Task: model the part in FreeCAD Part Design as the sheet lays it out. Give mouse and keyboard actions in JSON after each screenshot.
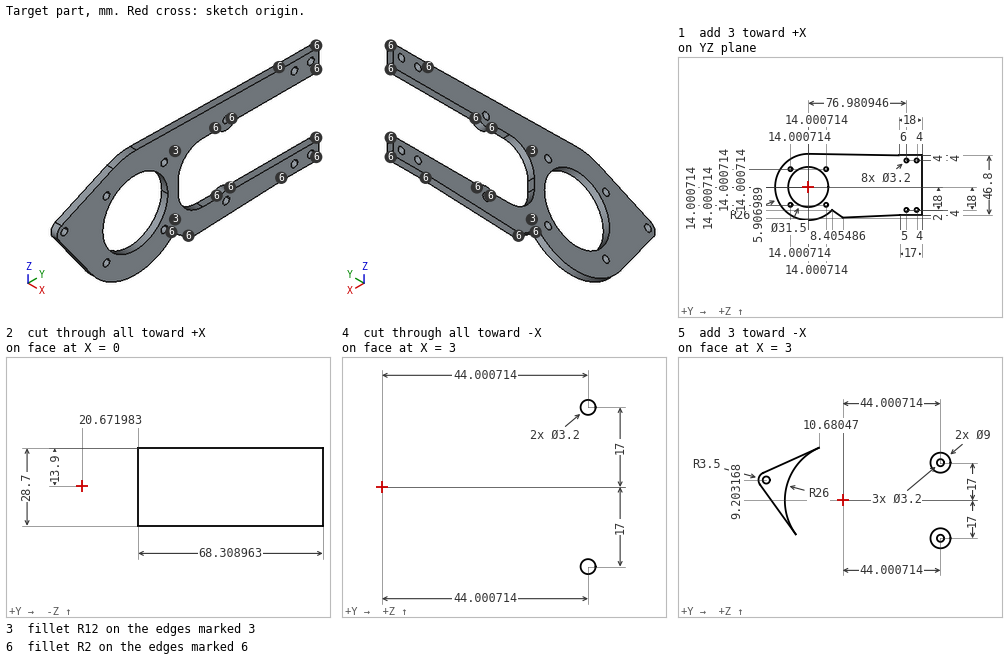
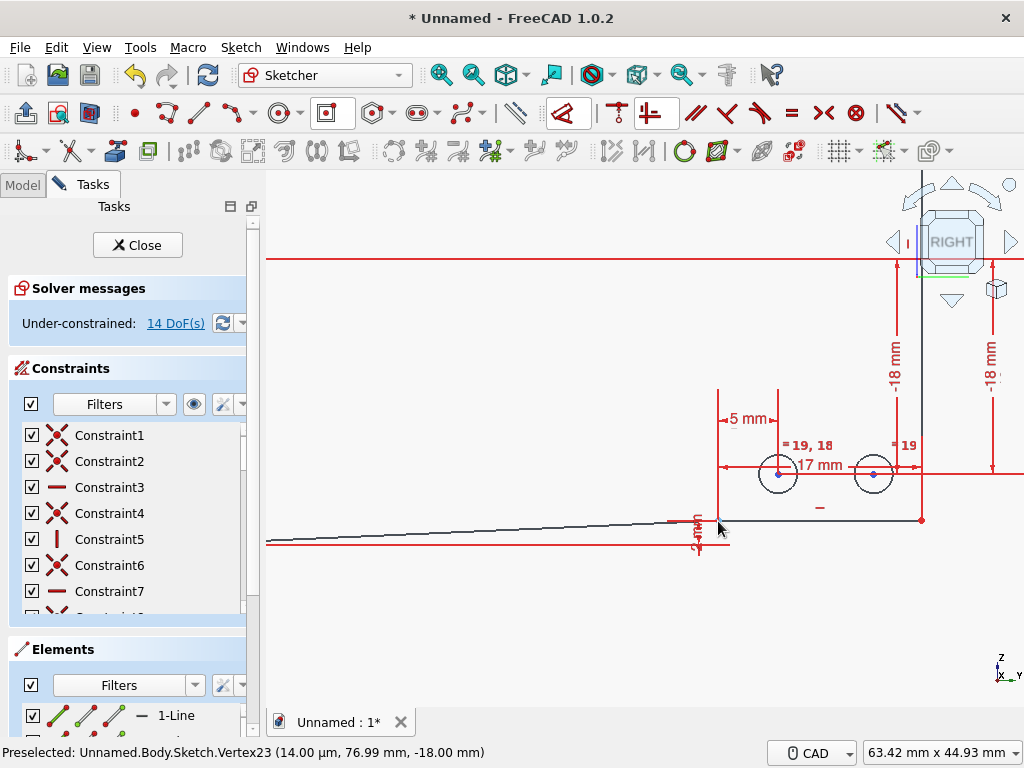
{"action": "left_click", "coordinate": [718, 521]}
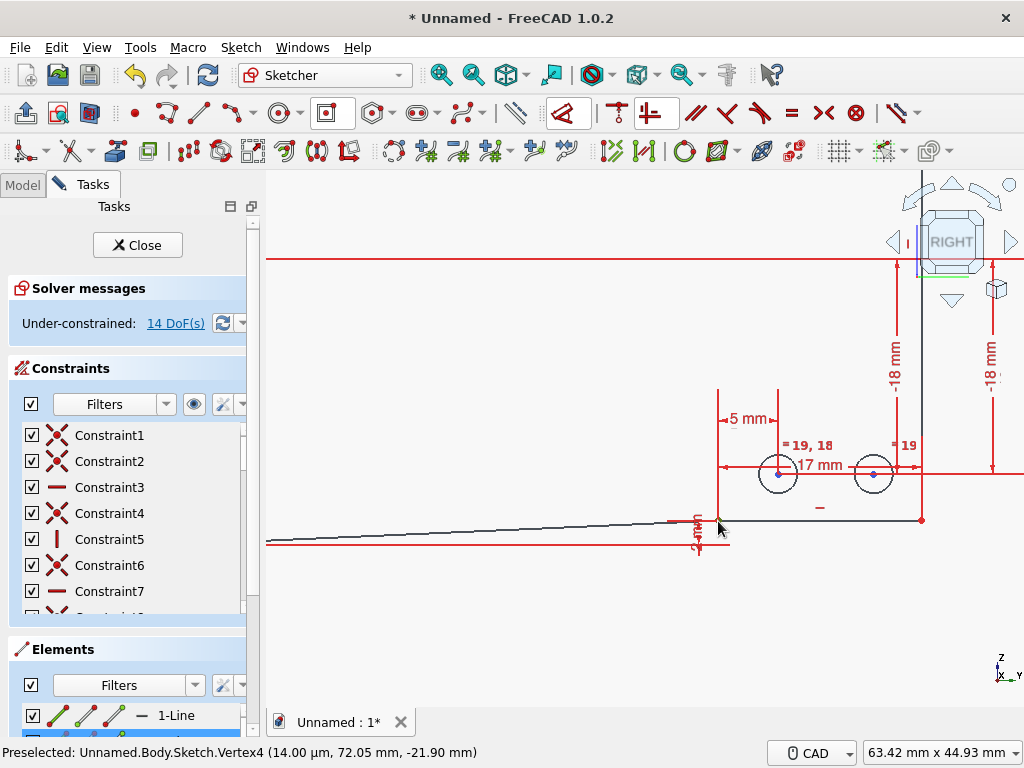
{"action": "left_click", "coordinate": [778, 474]}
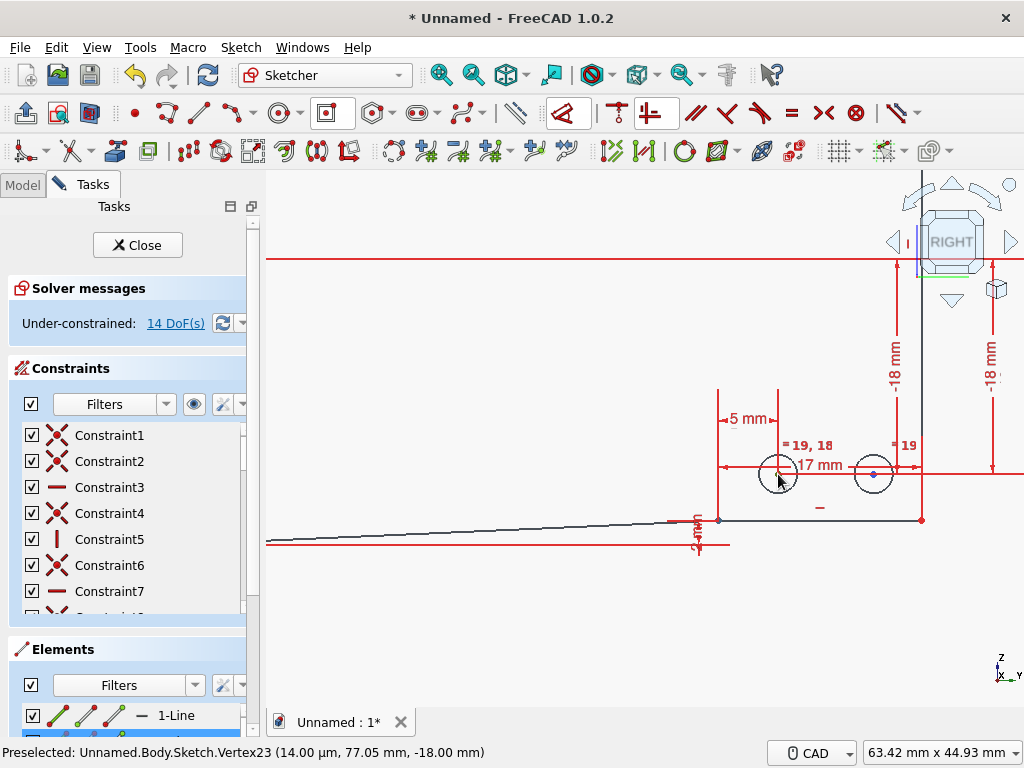
{"action": "left_click", "coordinate": [586, 114]}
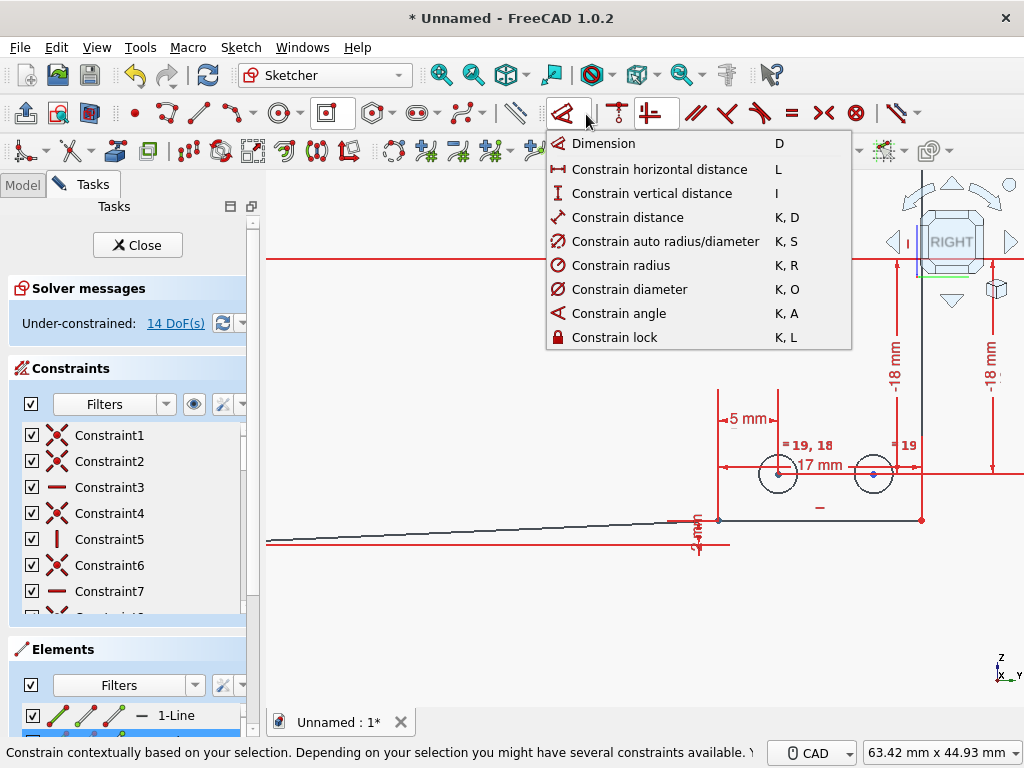
{"action": "left_click", "coordinate": [699, 193]}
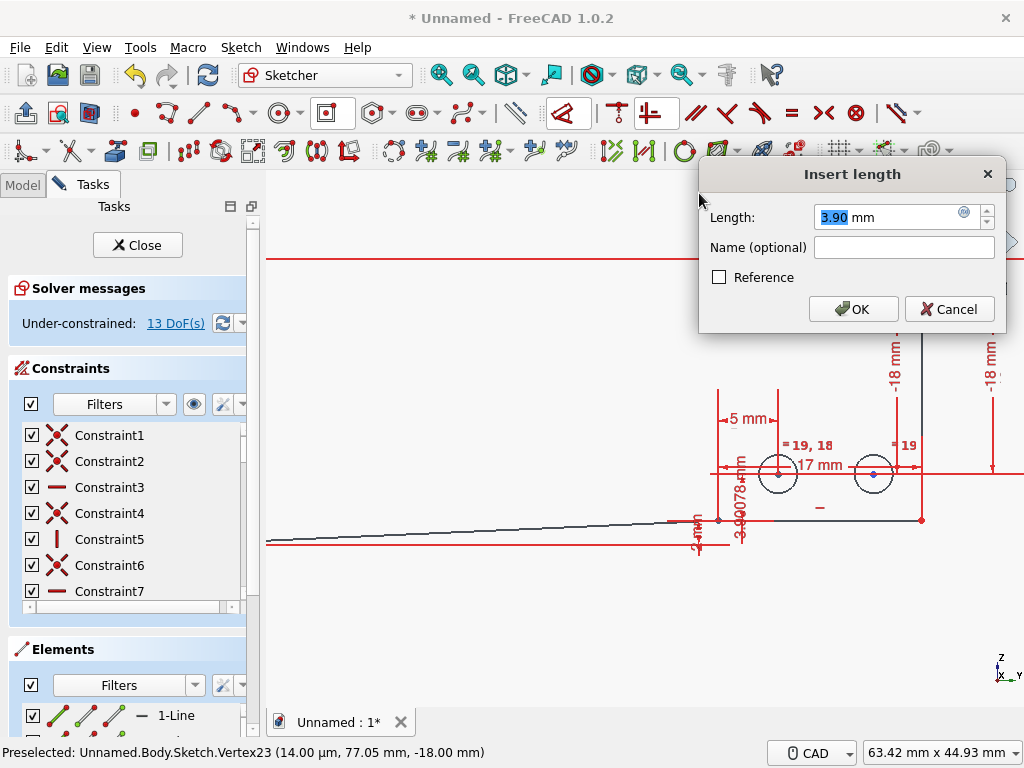
{"action": "type", "text": "4"}
{"action": "key", "text": "Return"}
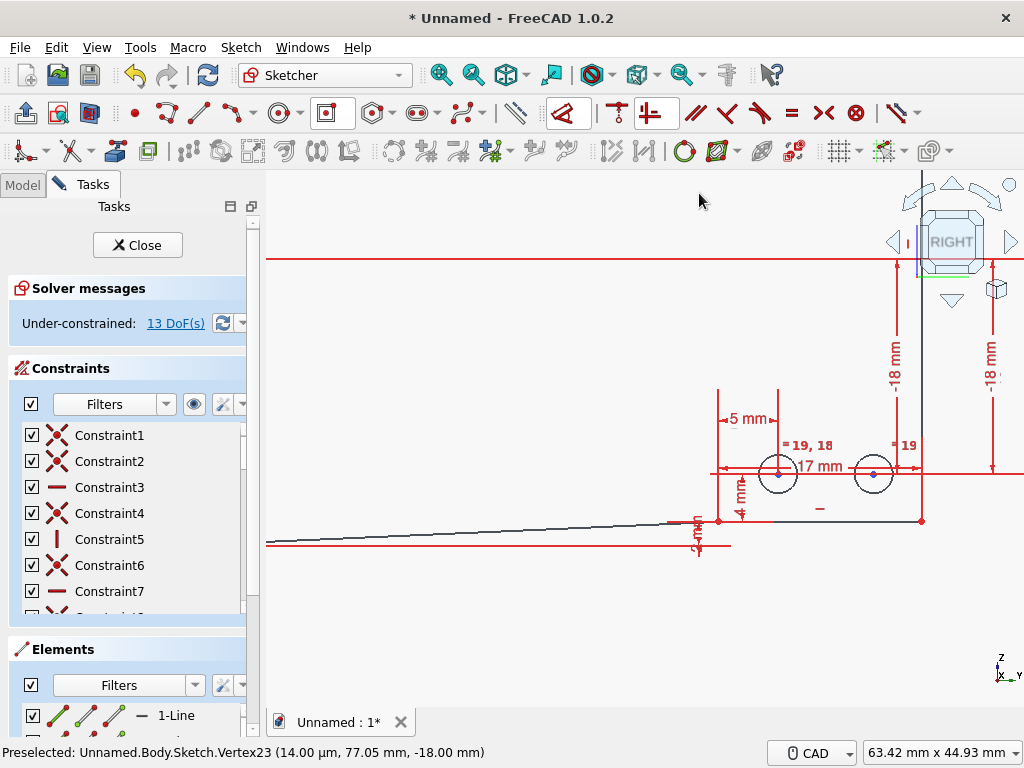
{"action": "scroll", "coordinate": [719, 521], "scroll_direction": "down", "scroll_amount": 6}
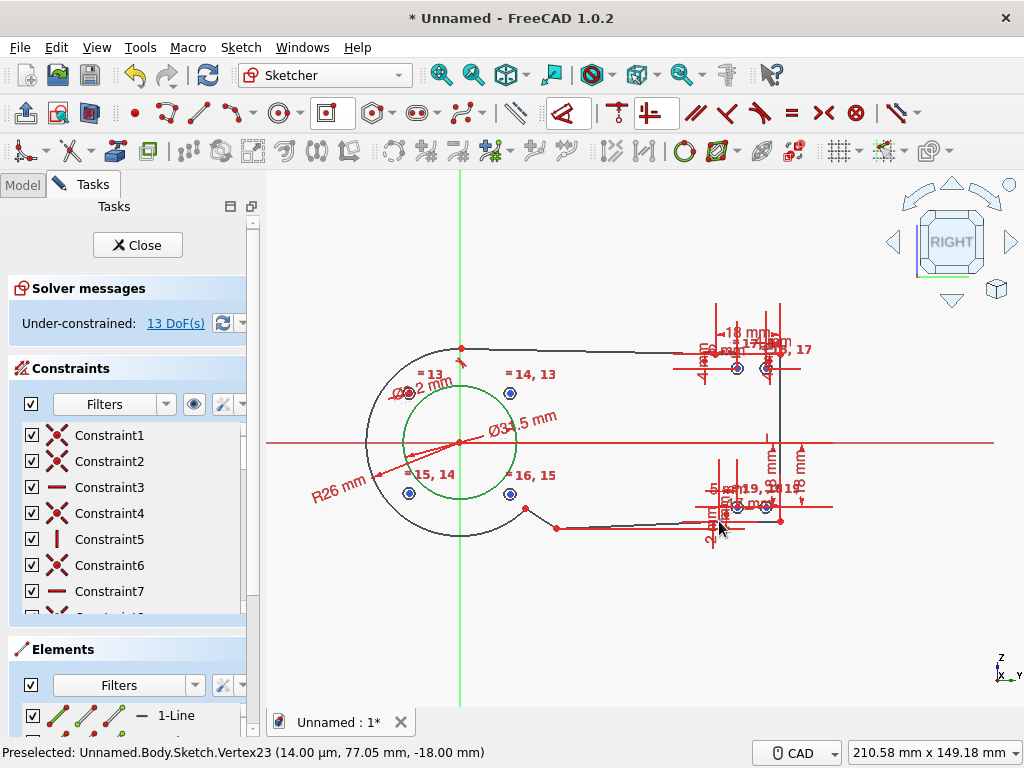
{"action": "scroll", "coordinate": [780, 522], "scroll_direction": "up", "scroll_amount": 6}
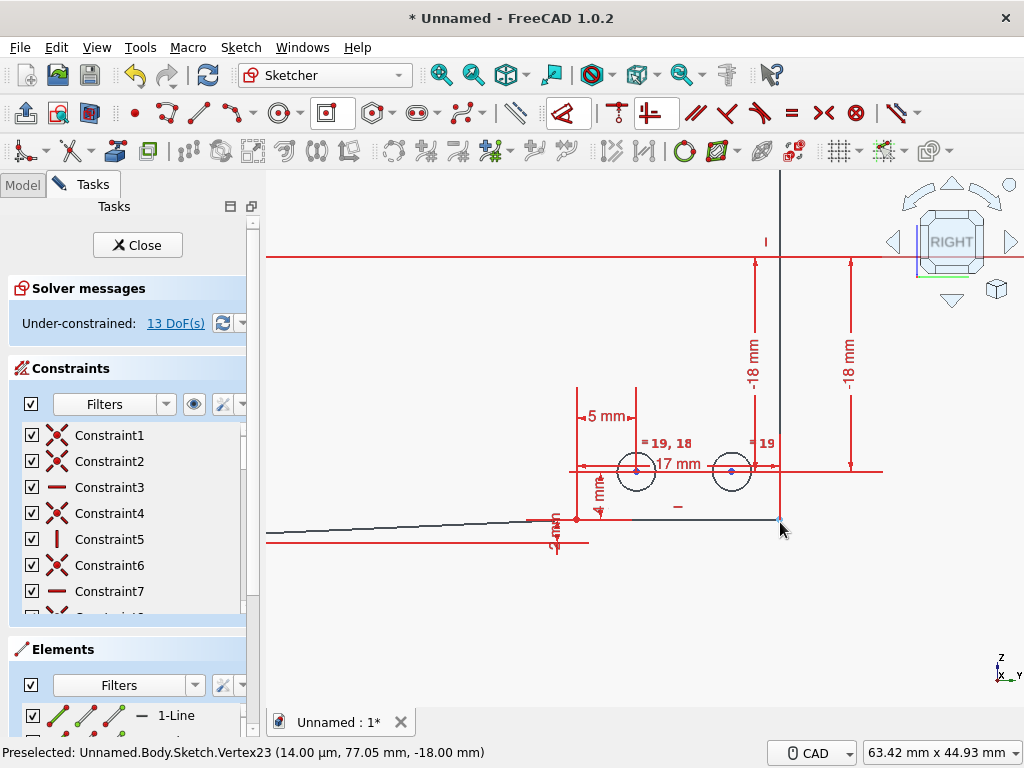
{"action": "left_click", "coordinate": [780, 520]}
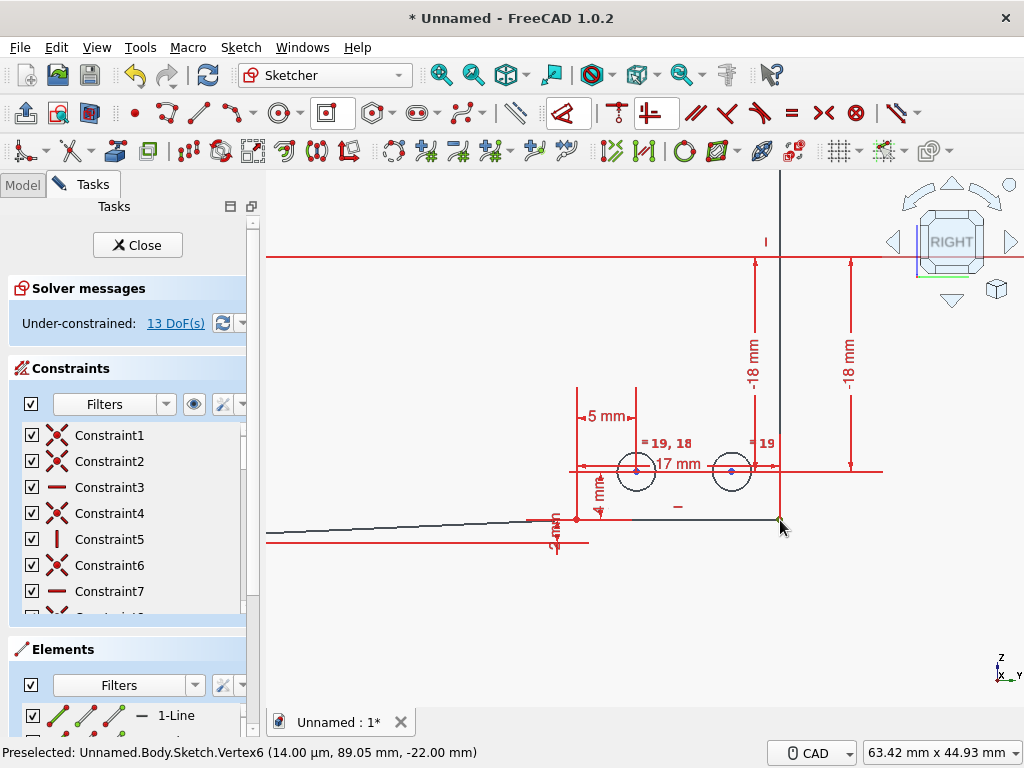
{"action": "left_click", "coordinate": [732, 472]}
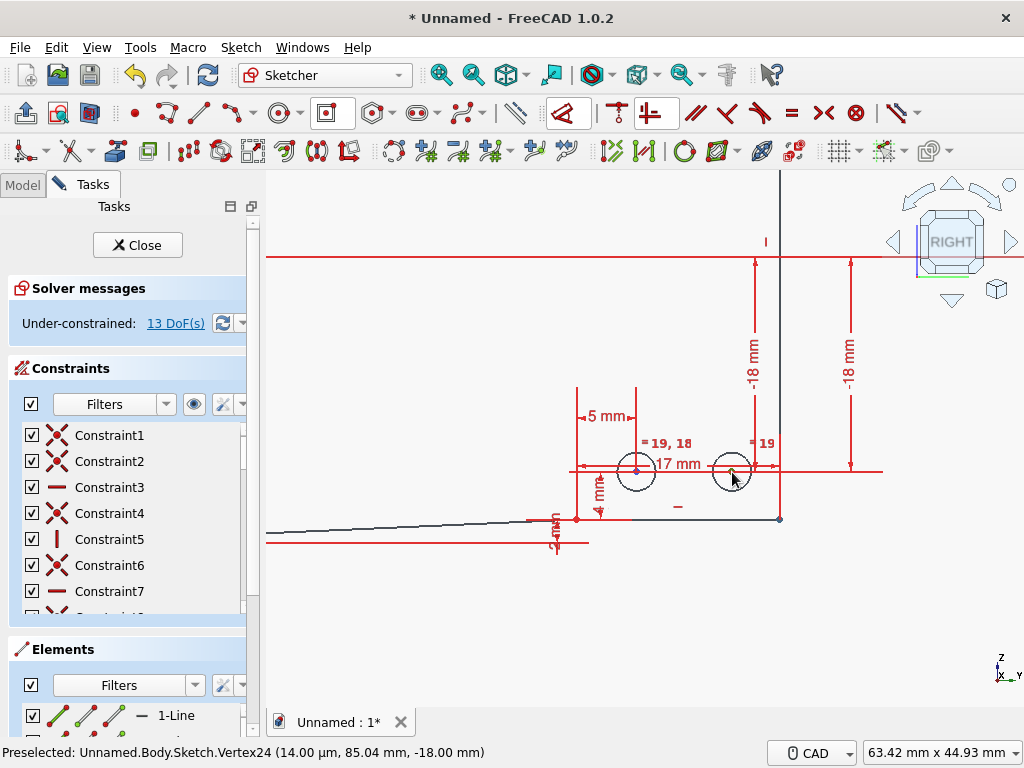
{"action": "key", "text": "l"}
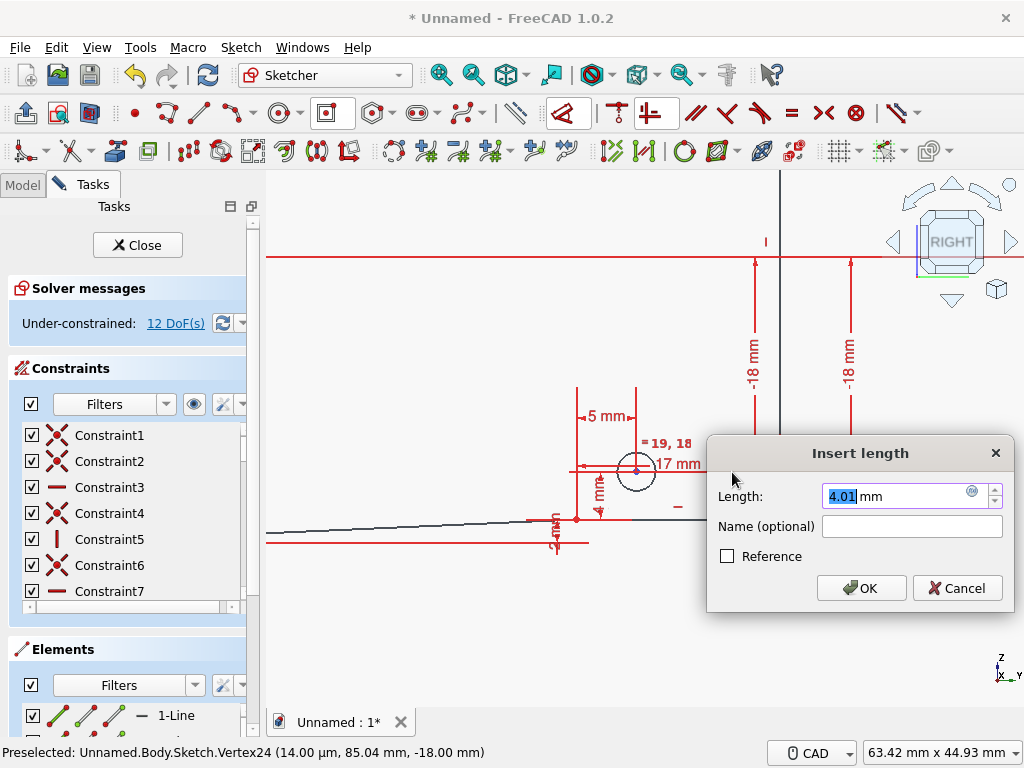
{"action": "type", "text": "4"}
{"action": "key", "text": "Return"}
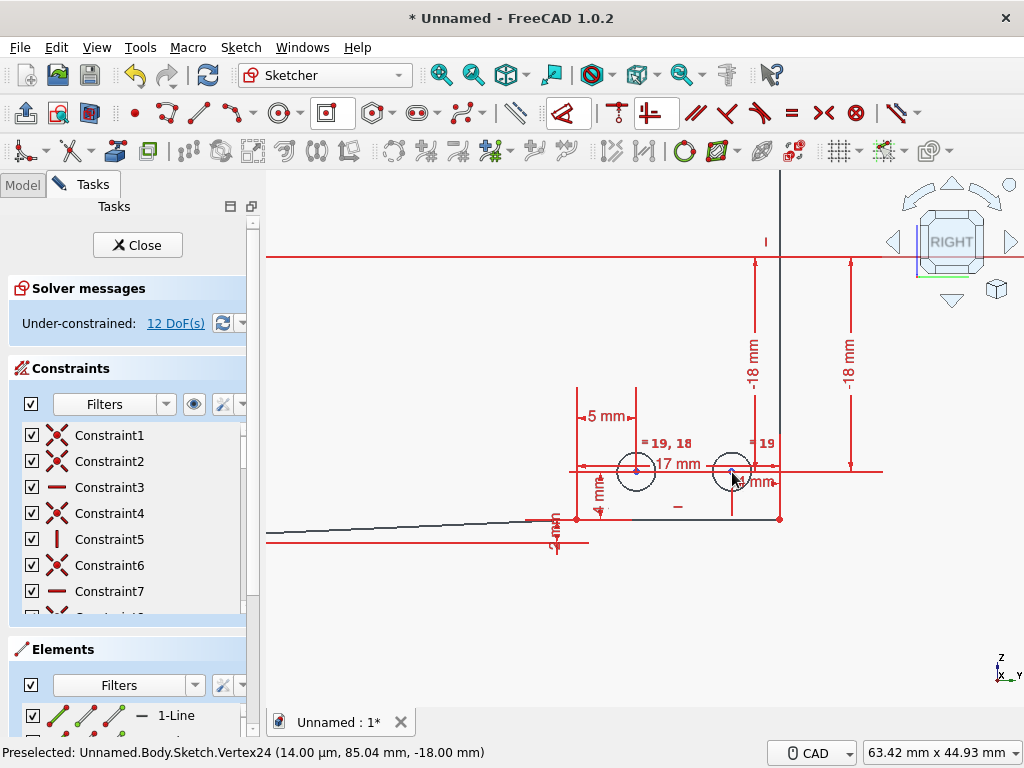
{"action": "scroll", "coordinate": [780, 522], "scroll_direction": "down", "scroll_amount": 6}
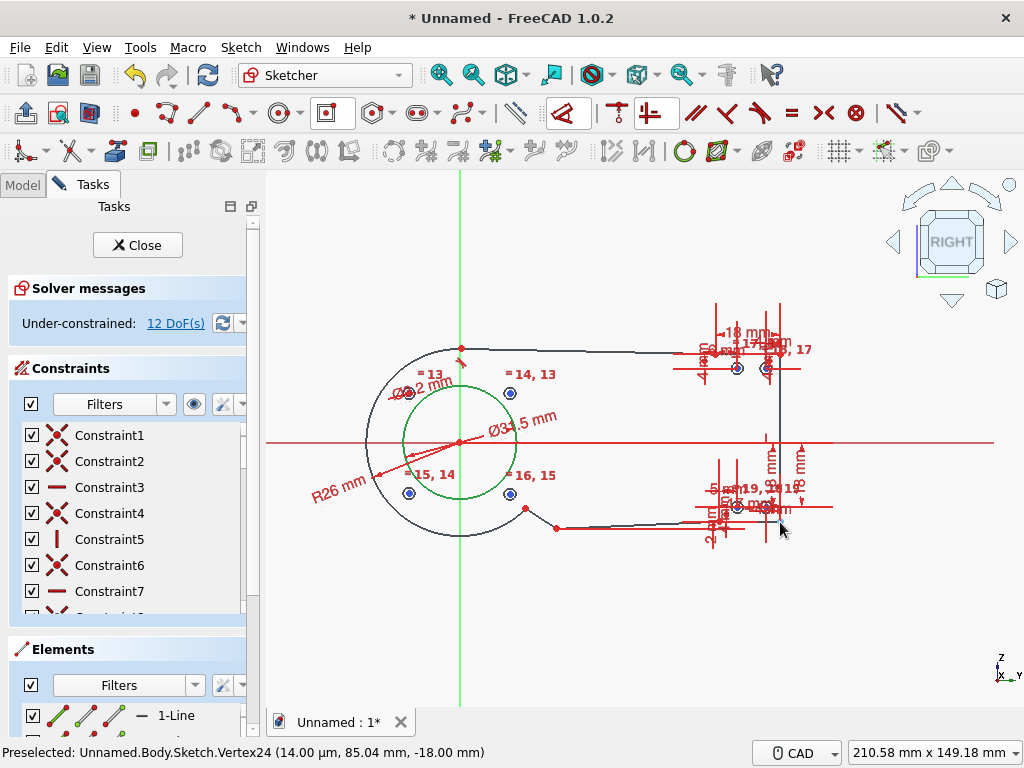
{"action": "left_click", "coordinate": [780, 438]}